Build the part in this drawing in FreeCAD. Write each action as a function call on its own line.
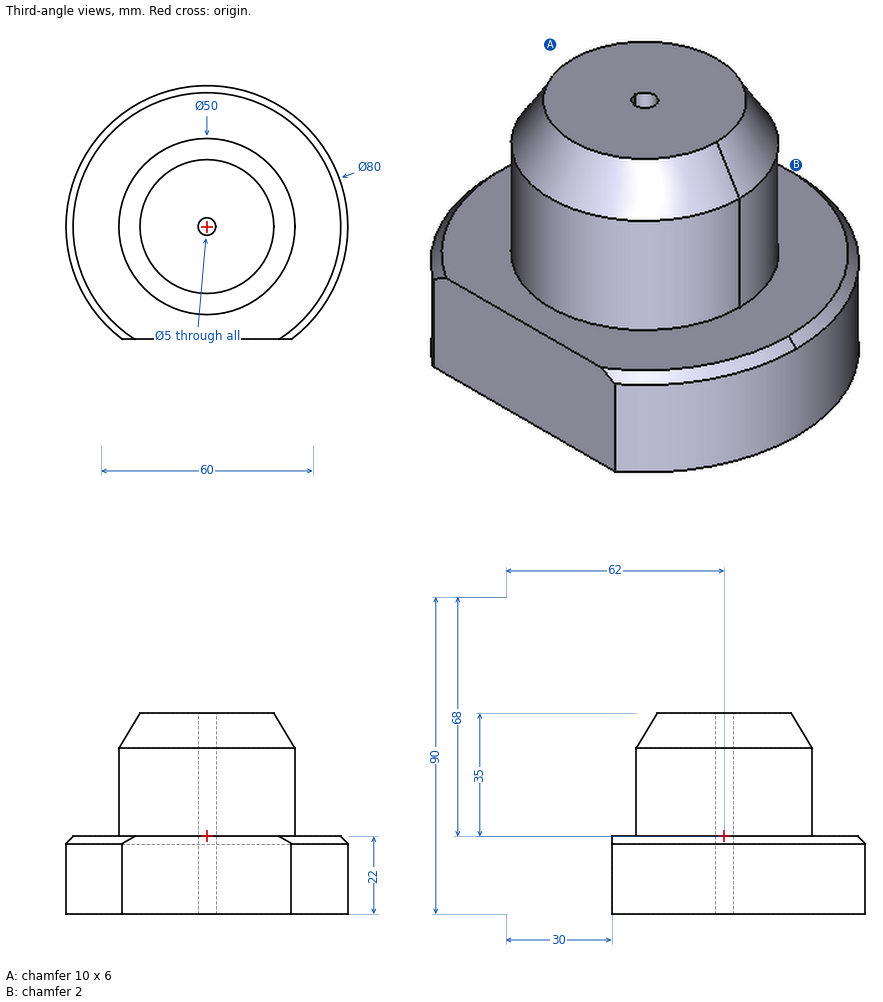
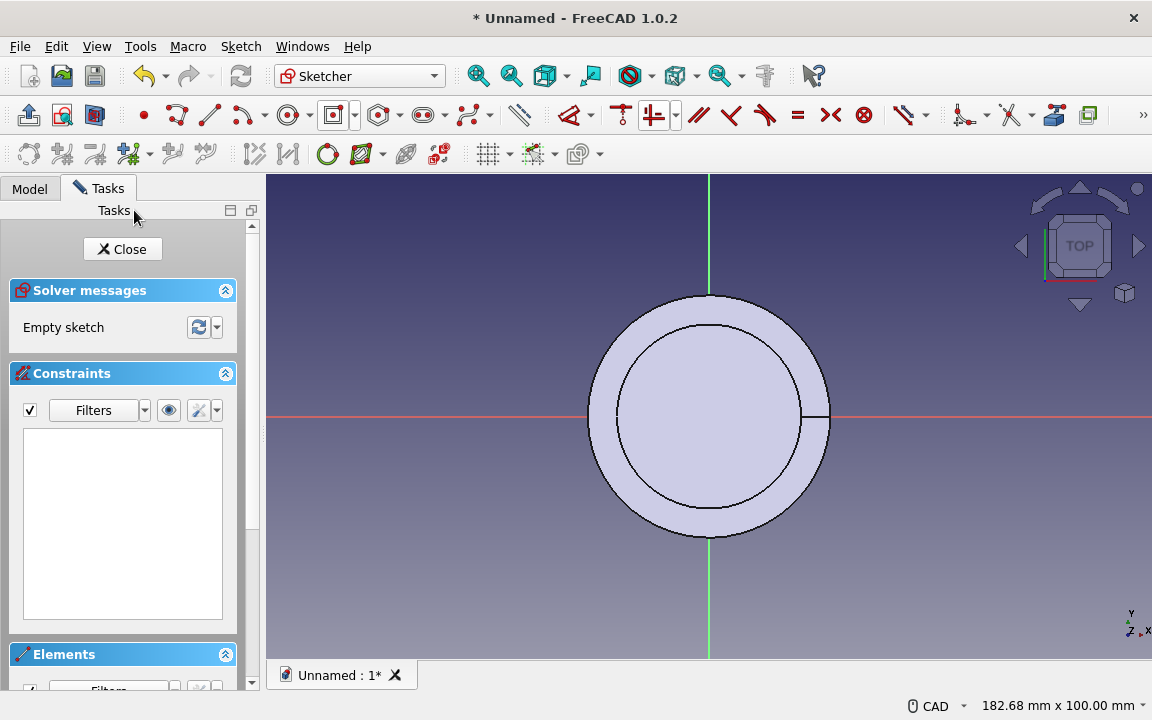
click(95, 116)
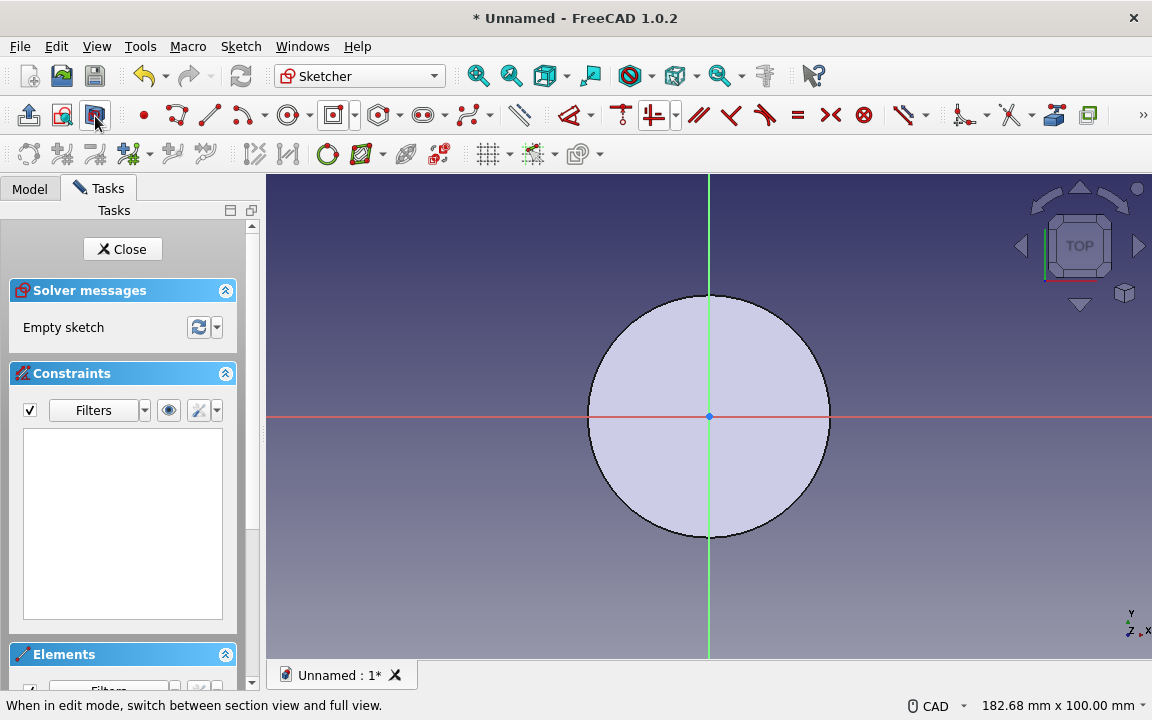
scroll(331, 416, down, 1)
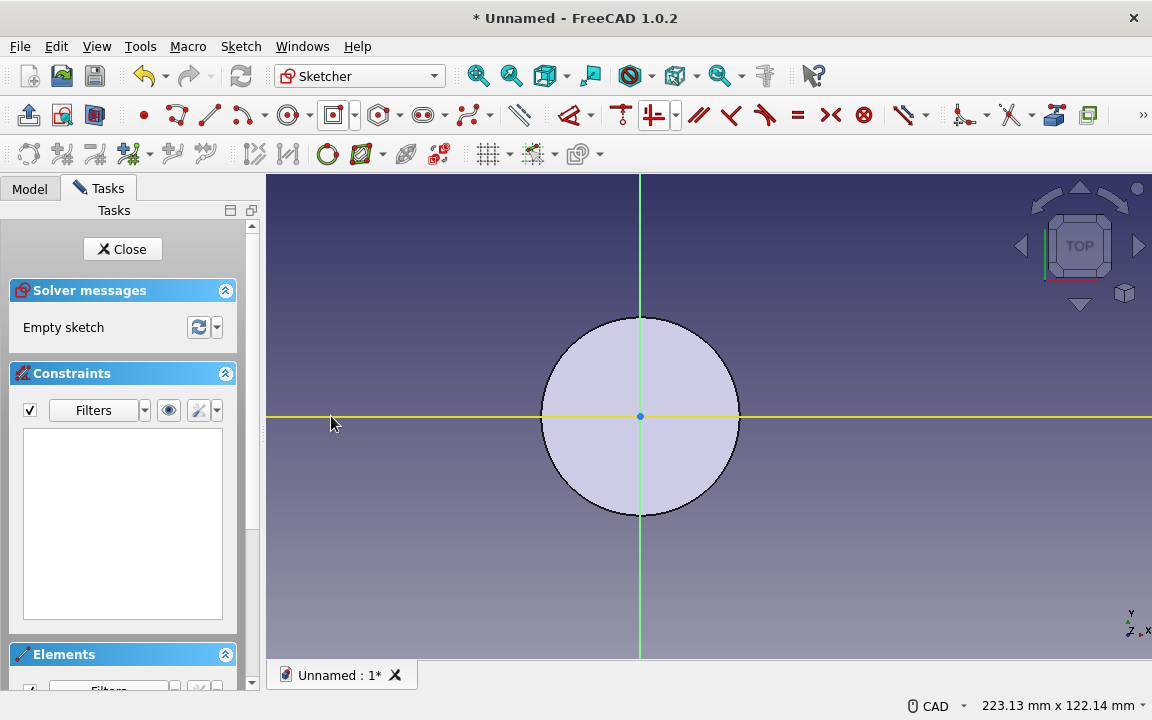
click(288, 116)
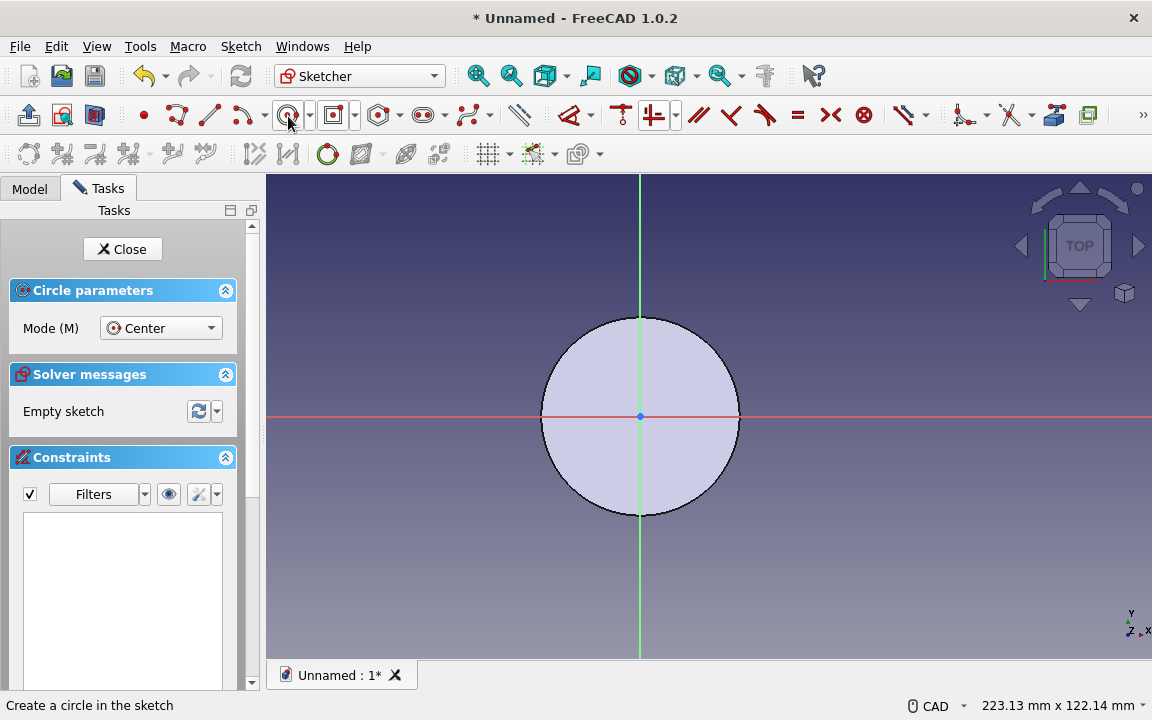
click(640, 416)
click(753, 304)
key(Escape)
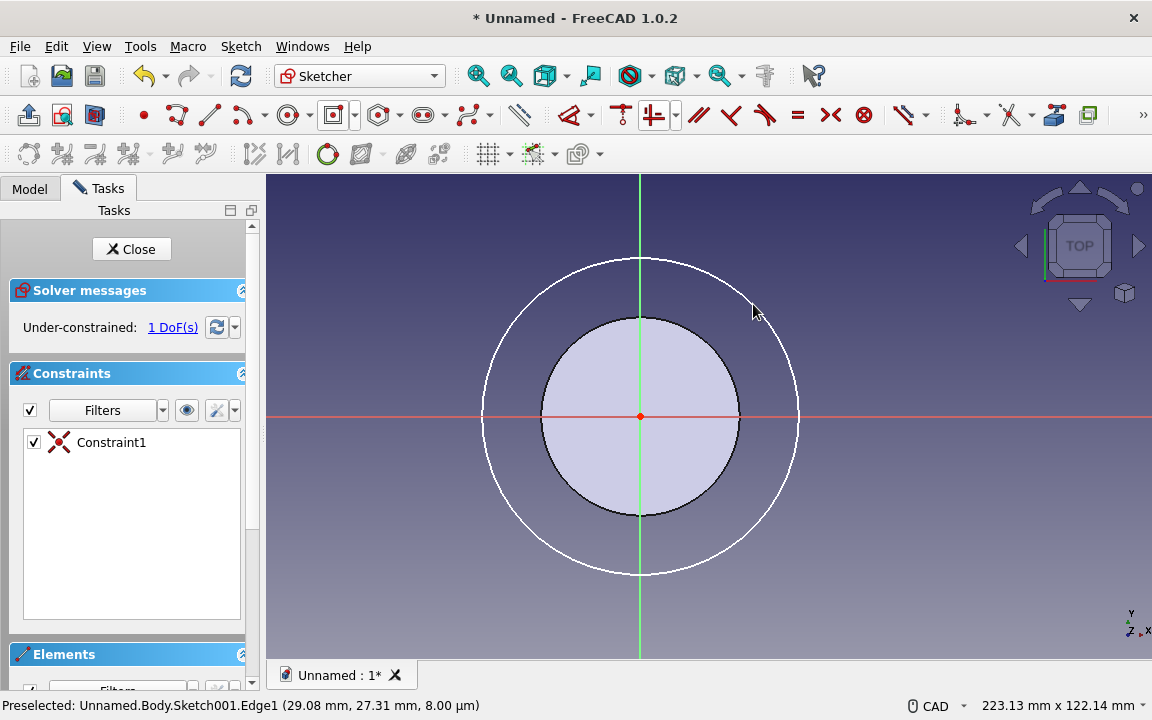
click(568, 116)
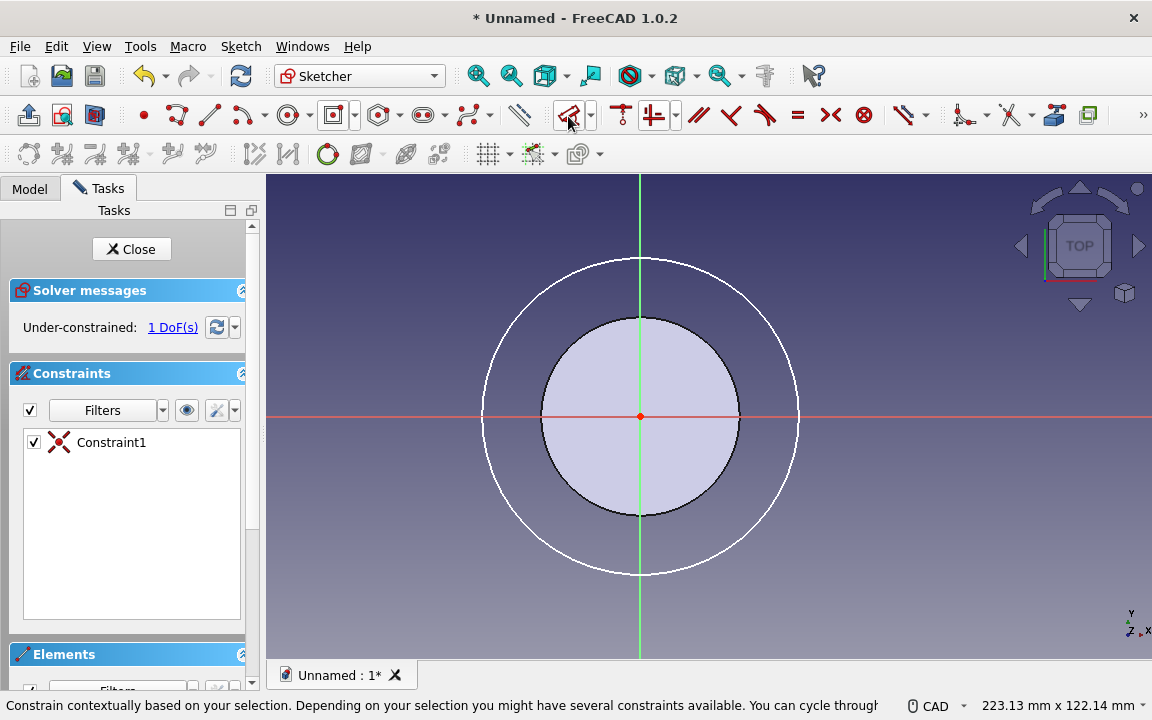
click(752, 304)
click(775, 281)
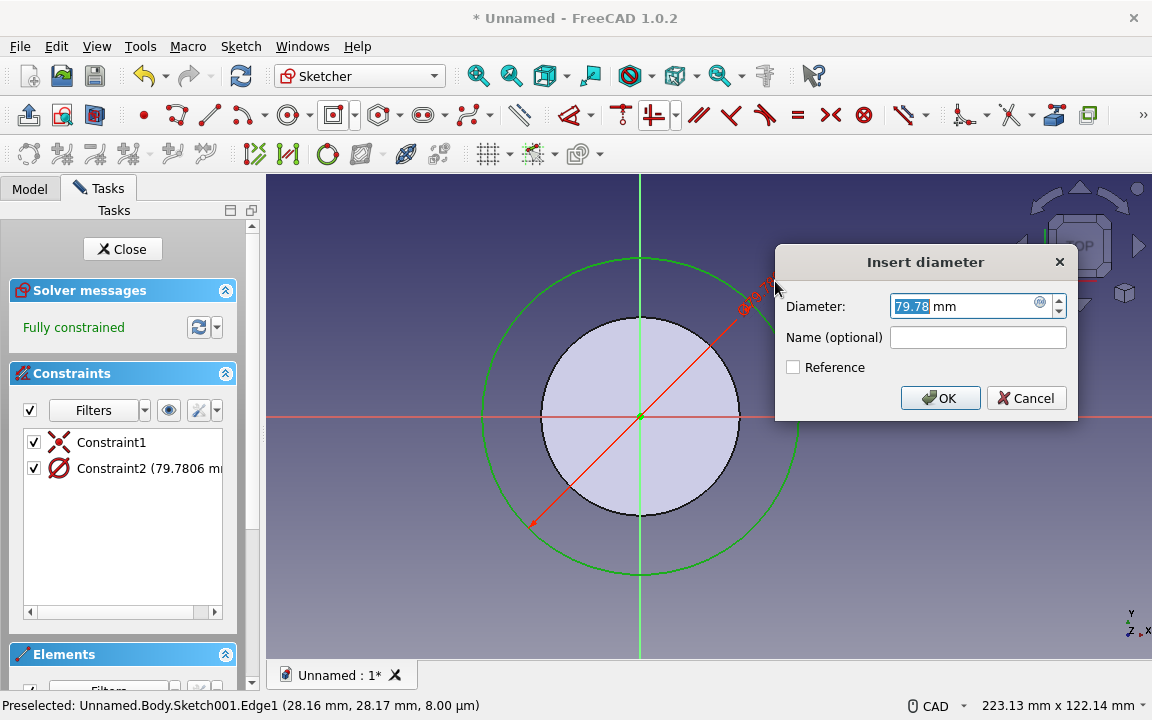
text(80)
key(Return)
key(Escape)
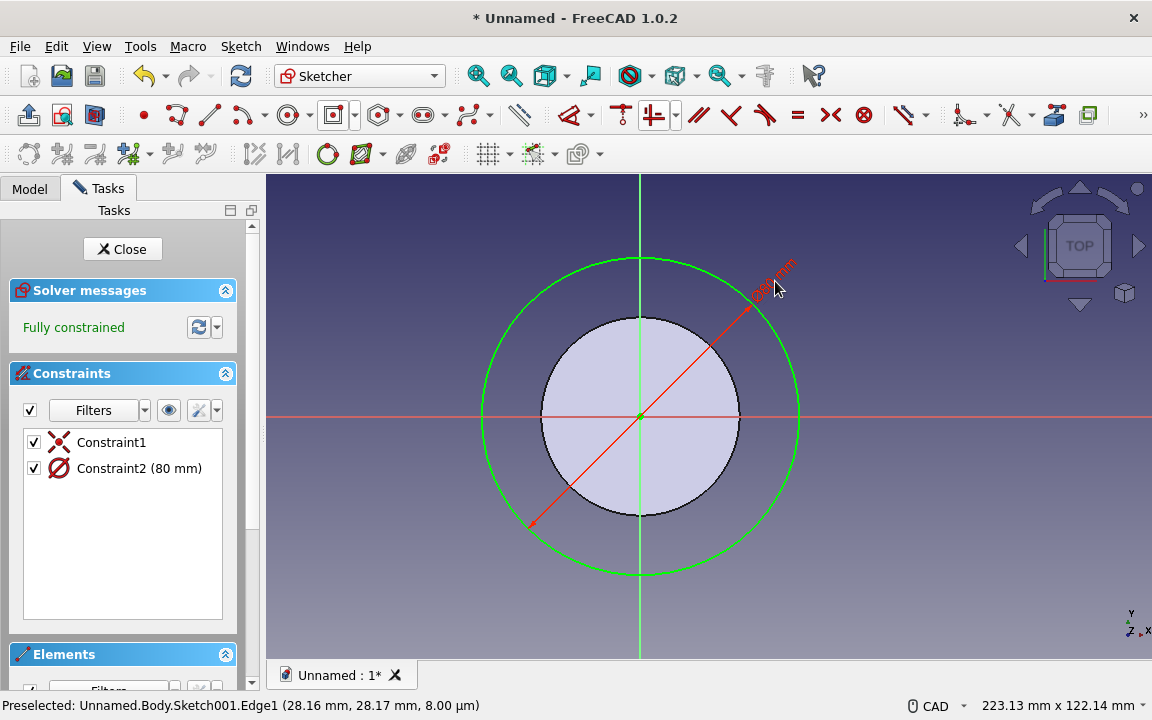
click(123, 249)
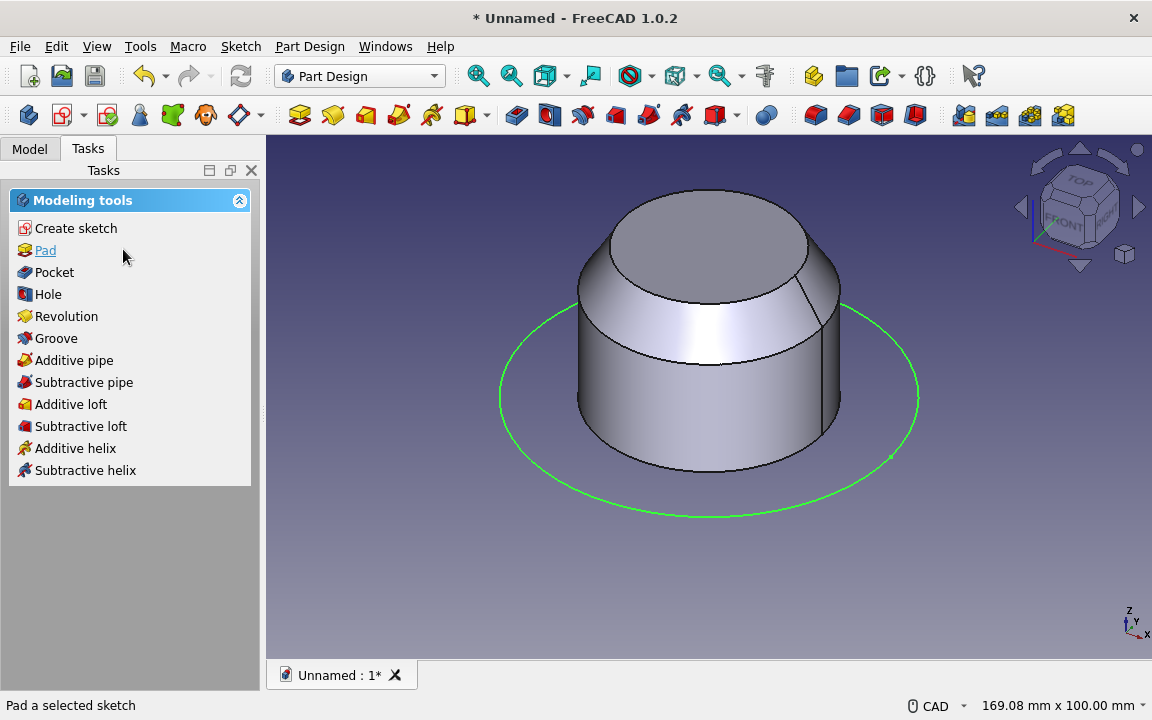
click(300, 116)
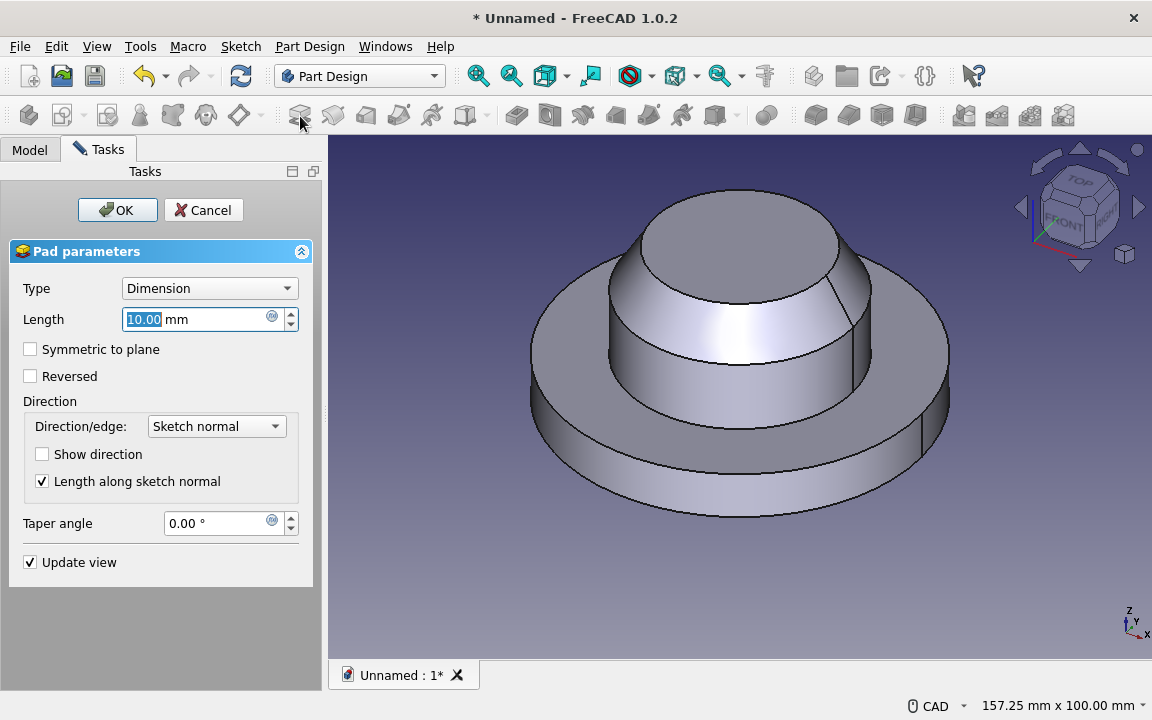
text(22)
key(Tab)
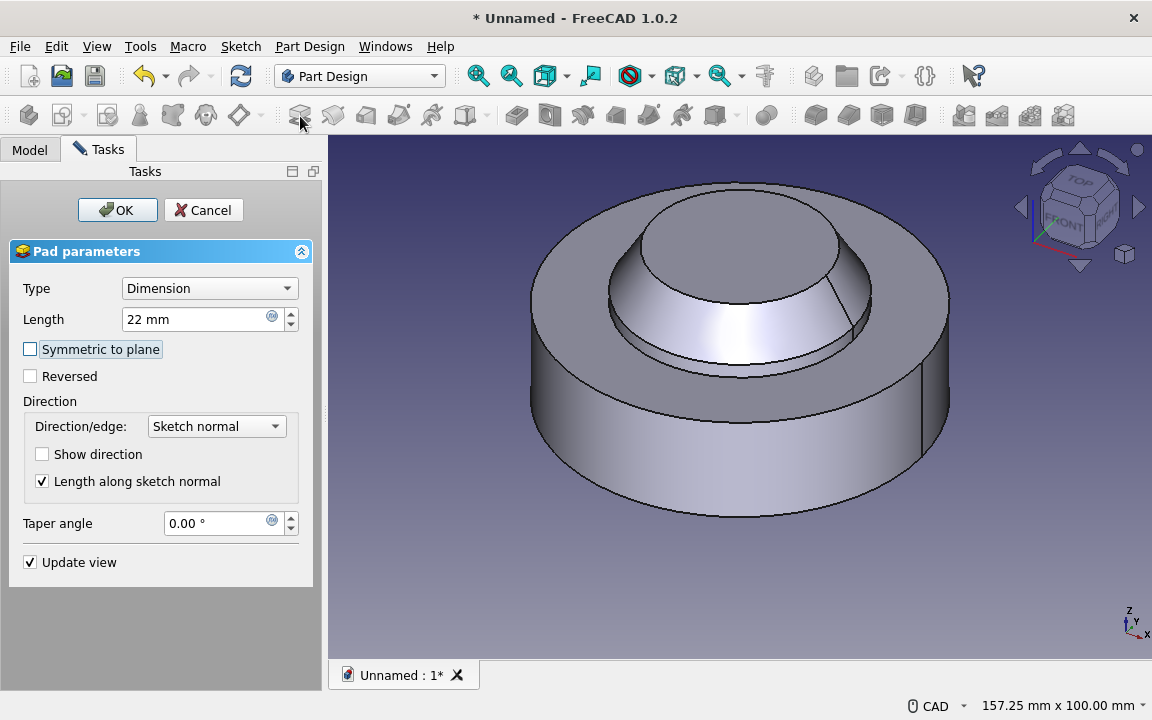
click(31, 376)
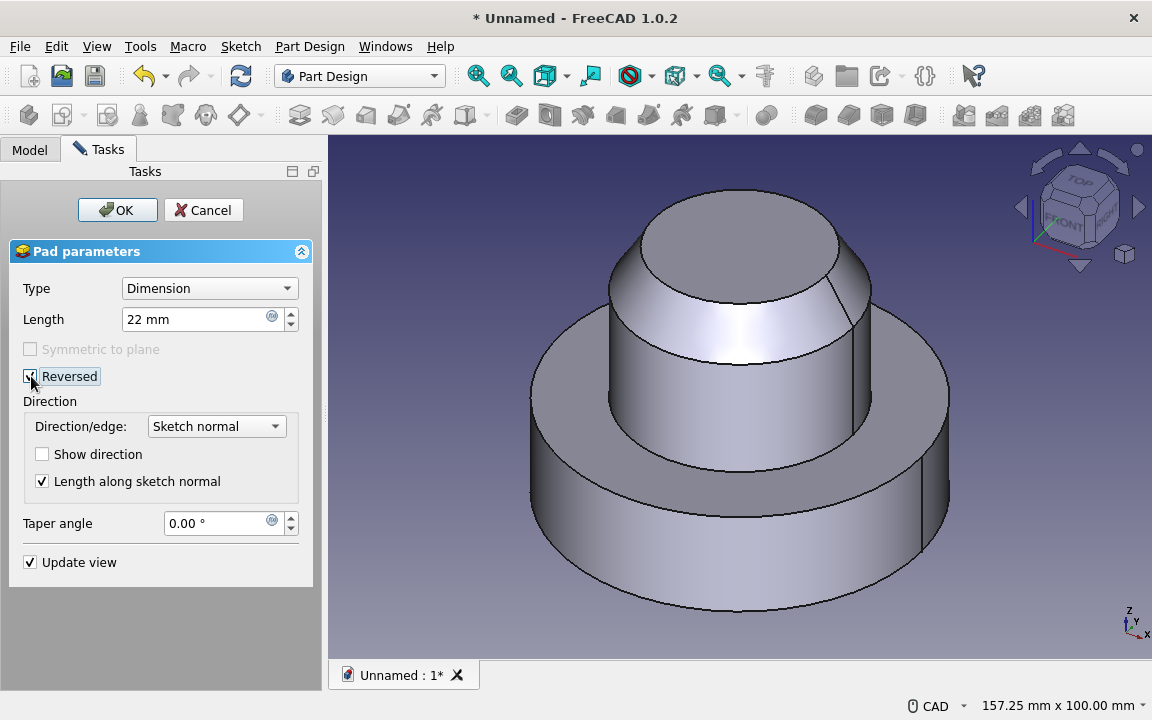
click(118, 210)